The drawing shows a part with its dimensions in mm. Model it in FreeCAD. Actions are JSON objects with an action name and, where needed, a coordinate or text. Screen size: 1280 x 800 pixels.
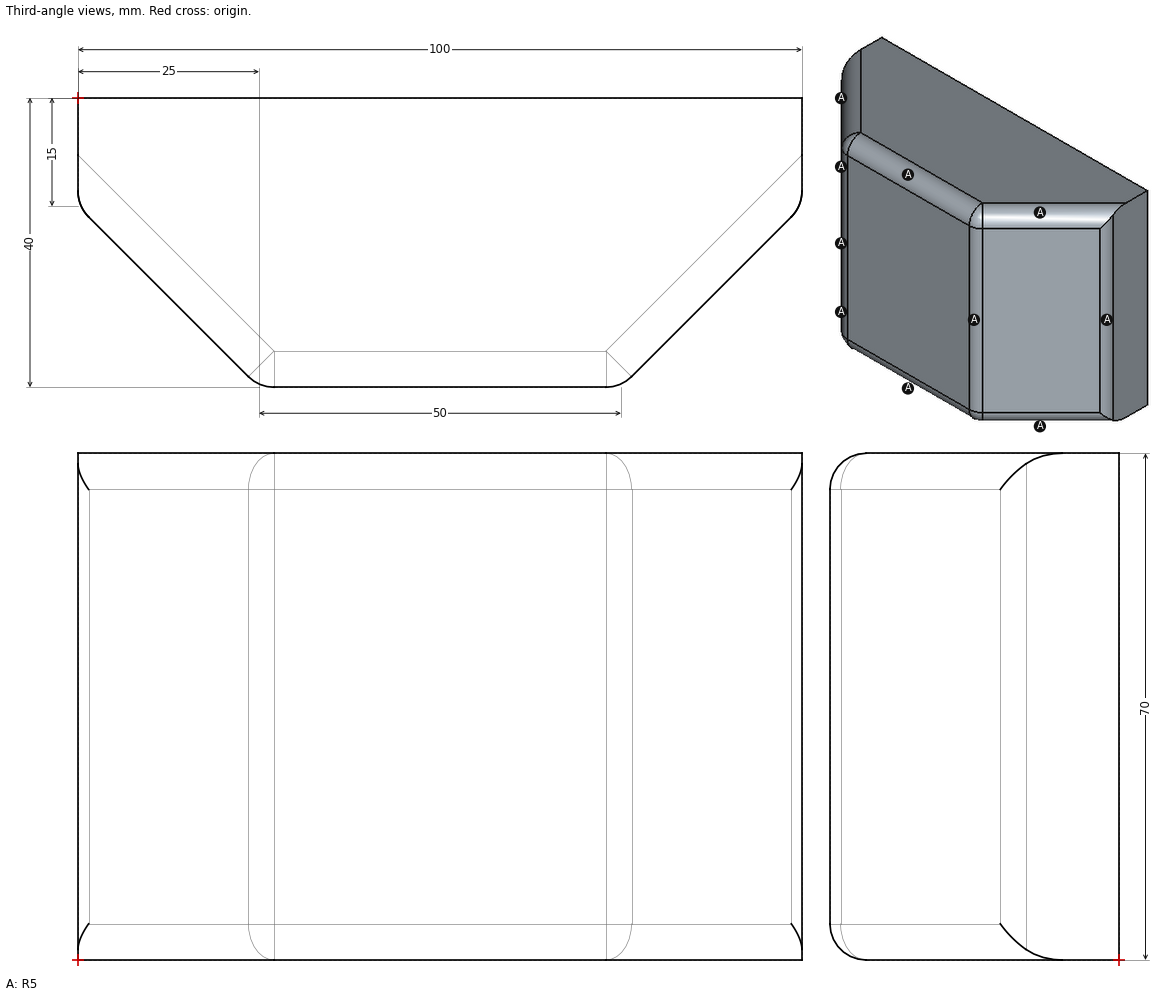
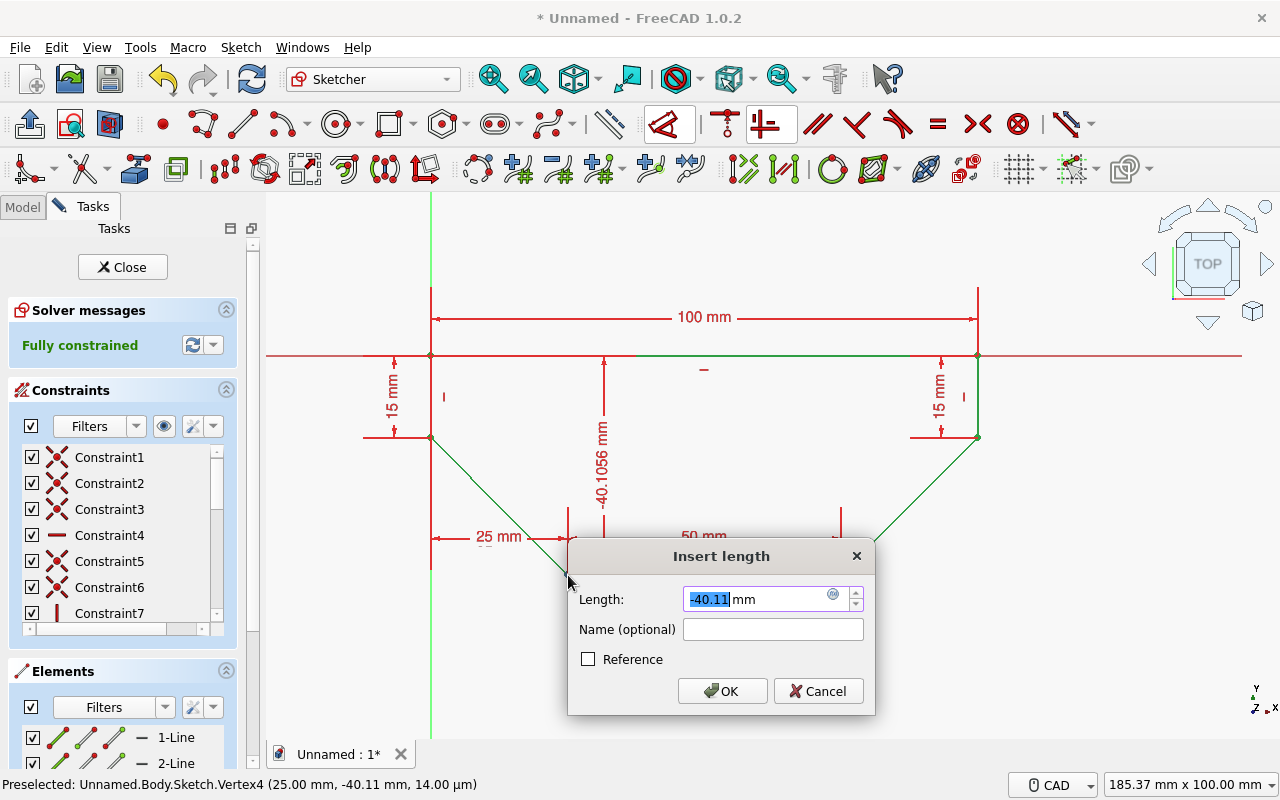
{"action": "type", "text": "-40"}
{"action": "key", "text": "Return"}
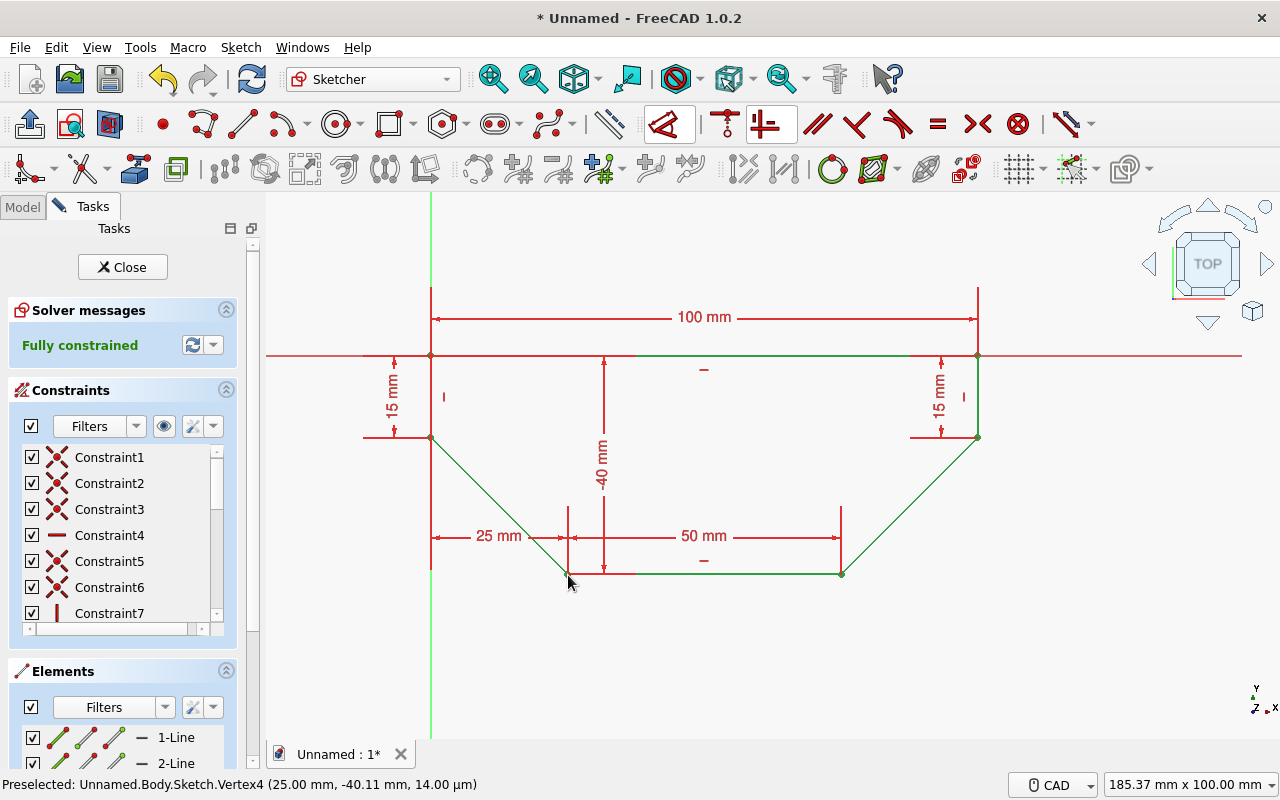
{"action": "left_click", "coordinate": [123, 267]}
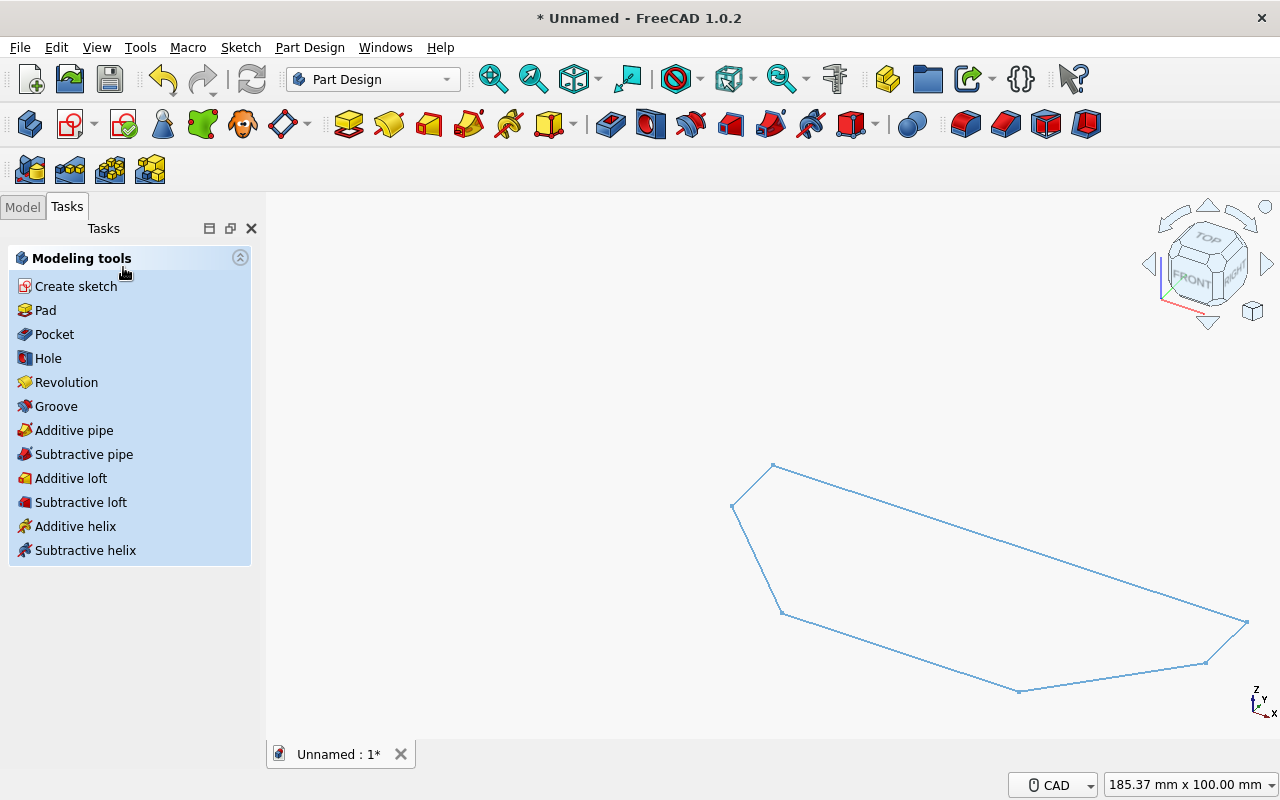
{"action": "left_click", "coordinate": [350, 124]}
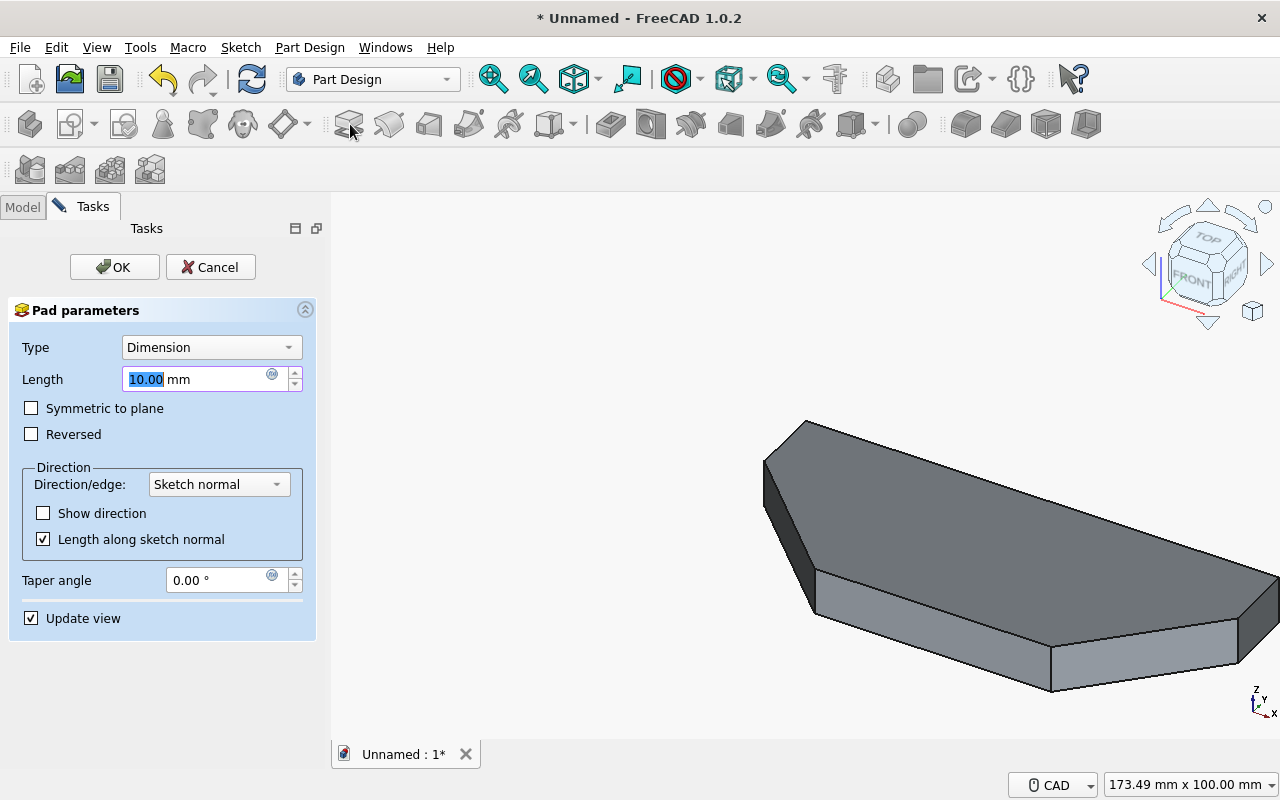
{"action": "type", "text": "70"}
{"action": "key", "text": "Tab"}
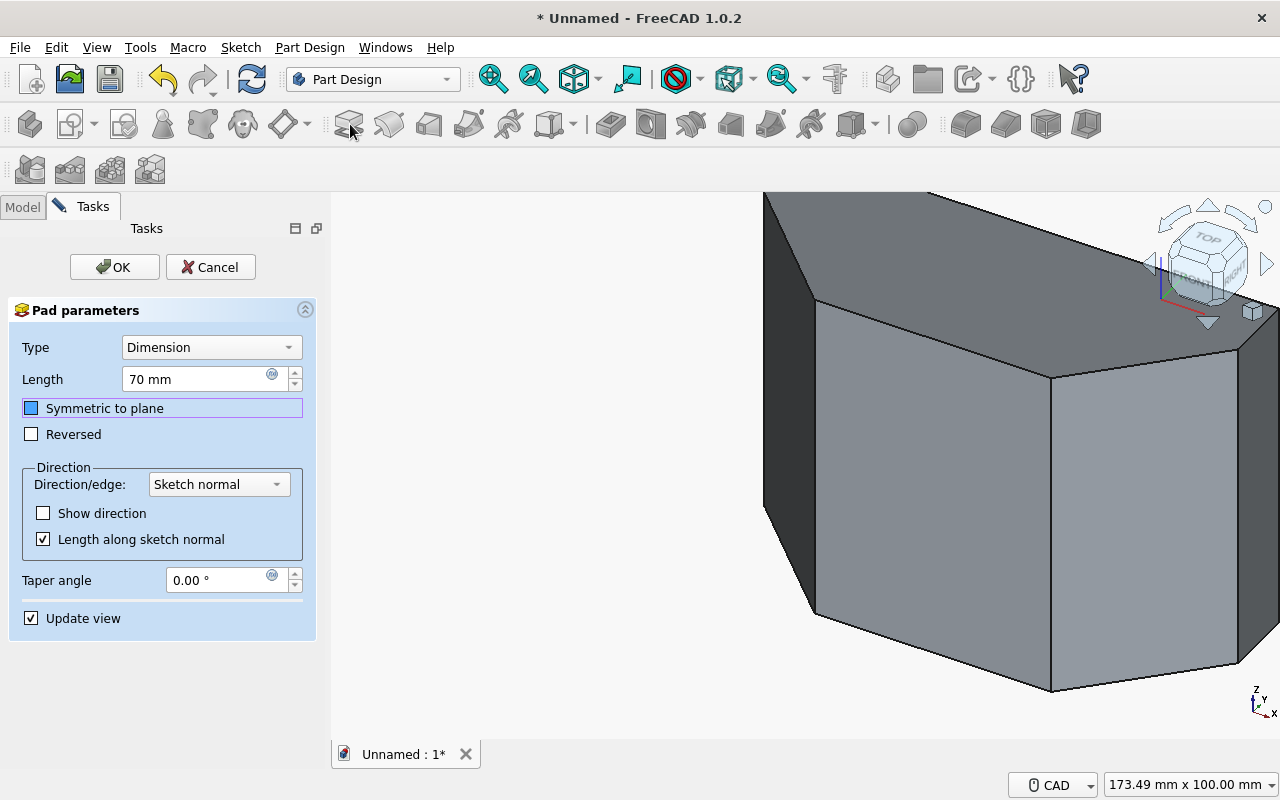
{"action": "left_click", "coordinate": [115, 267]}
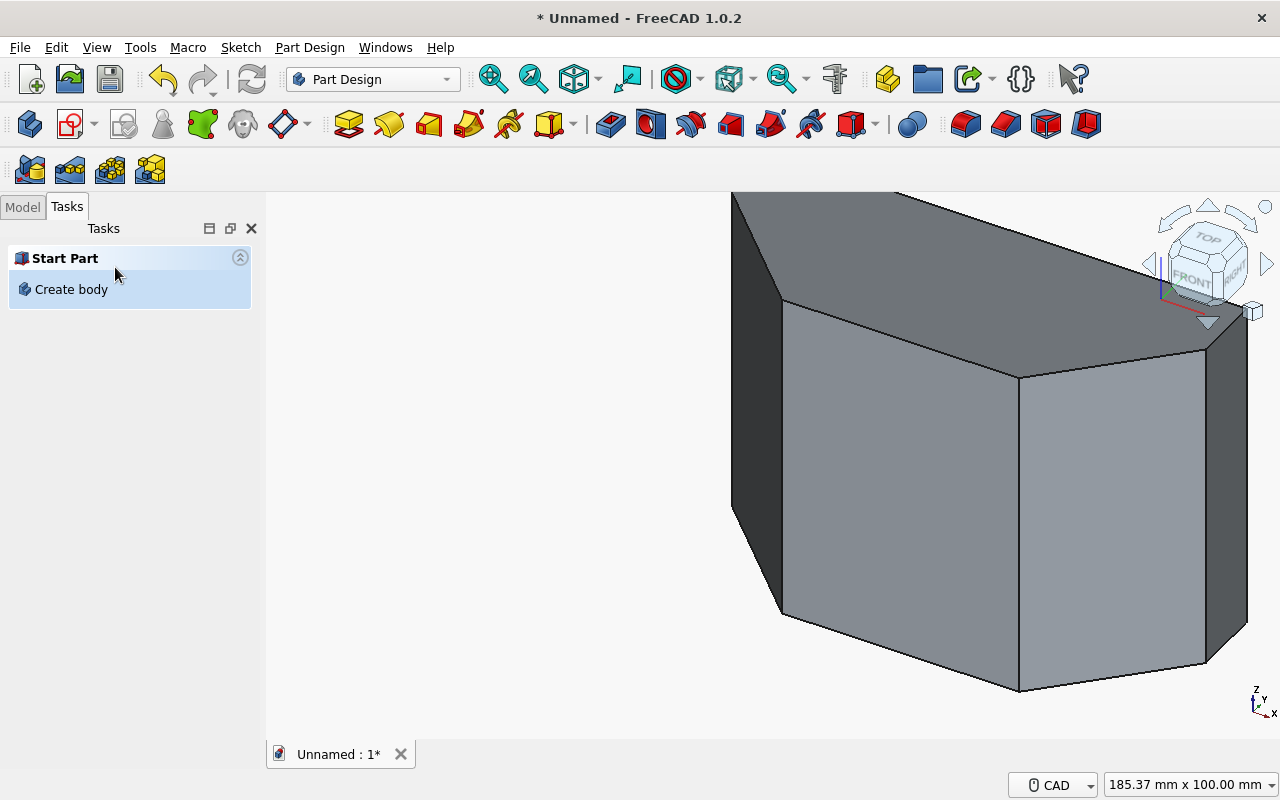
{"action": "left_click", "coordinate": [494, 80]}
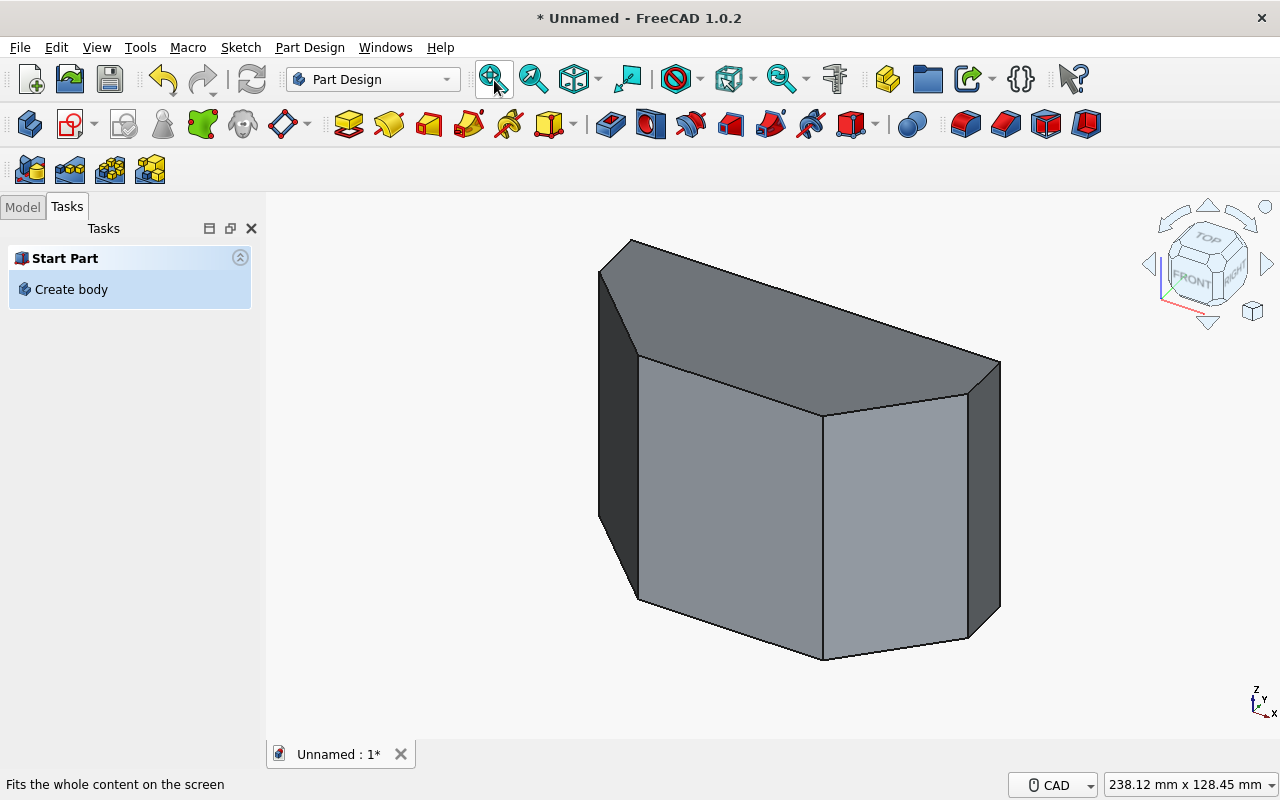
{"action": "left_click", "coordinate": [730, 472]}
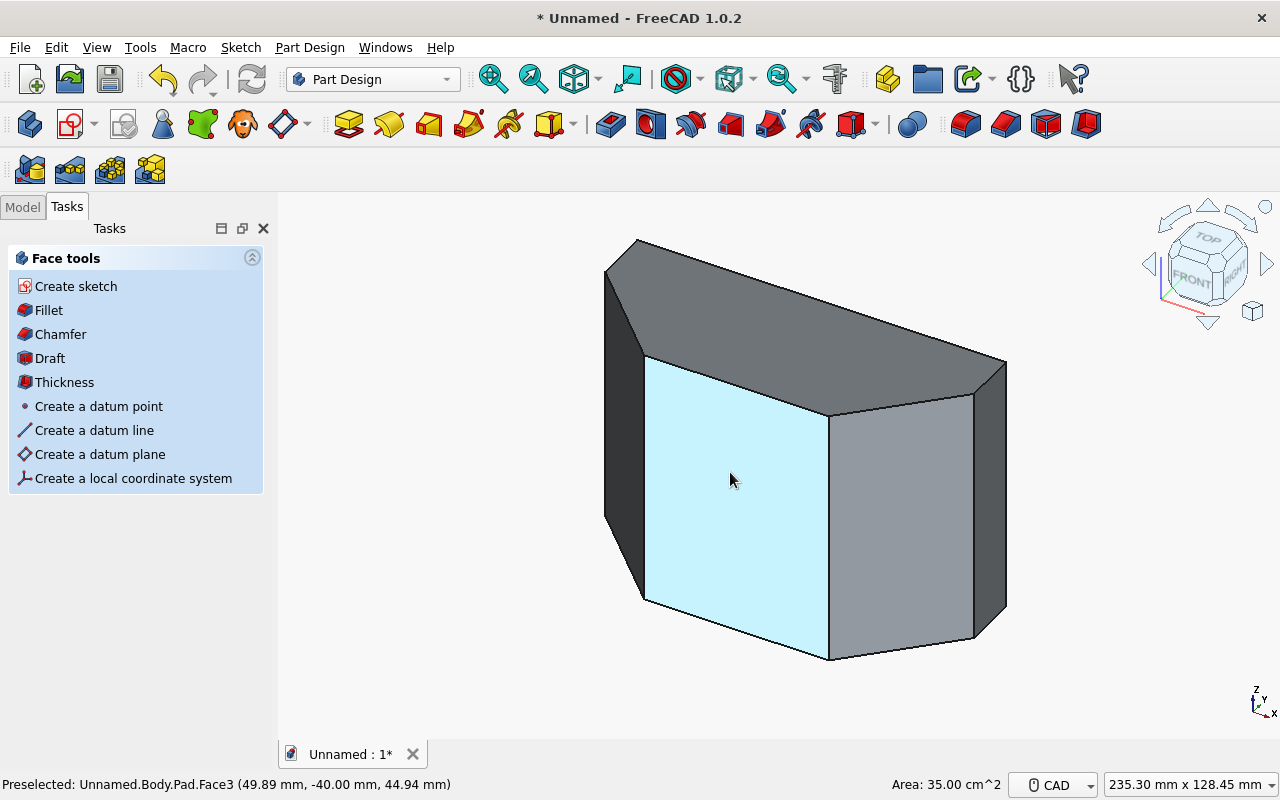
{"action": "left_click", "coordinate": [625, 400], "text": "ctrl"}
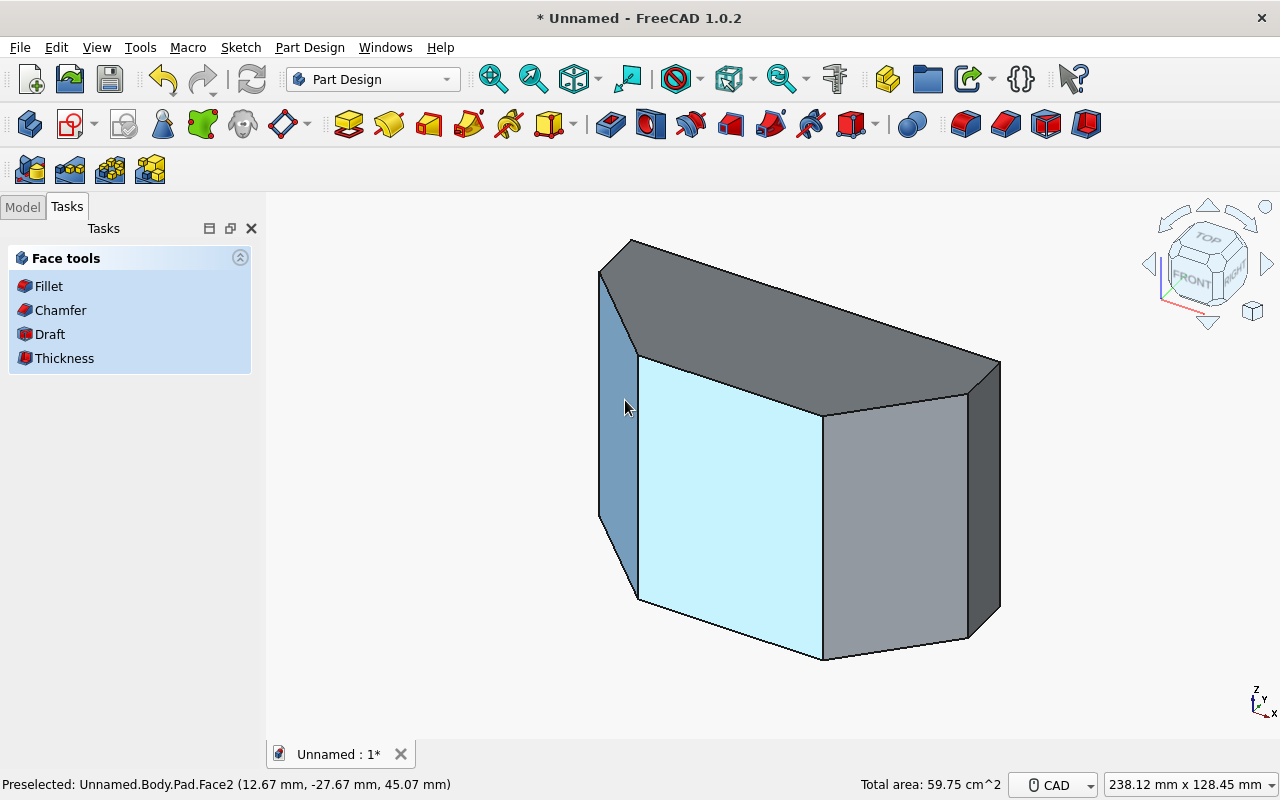
{"action": "left_click", "coordinate": [895, 491], "text": "ctrl"}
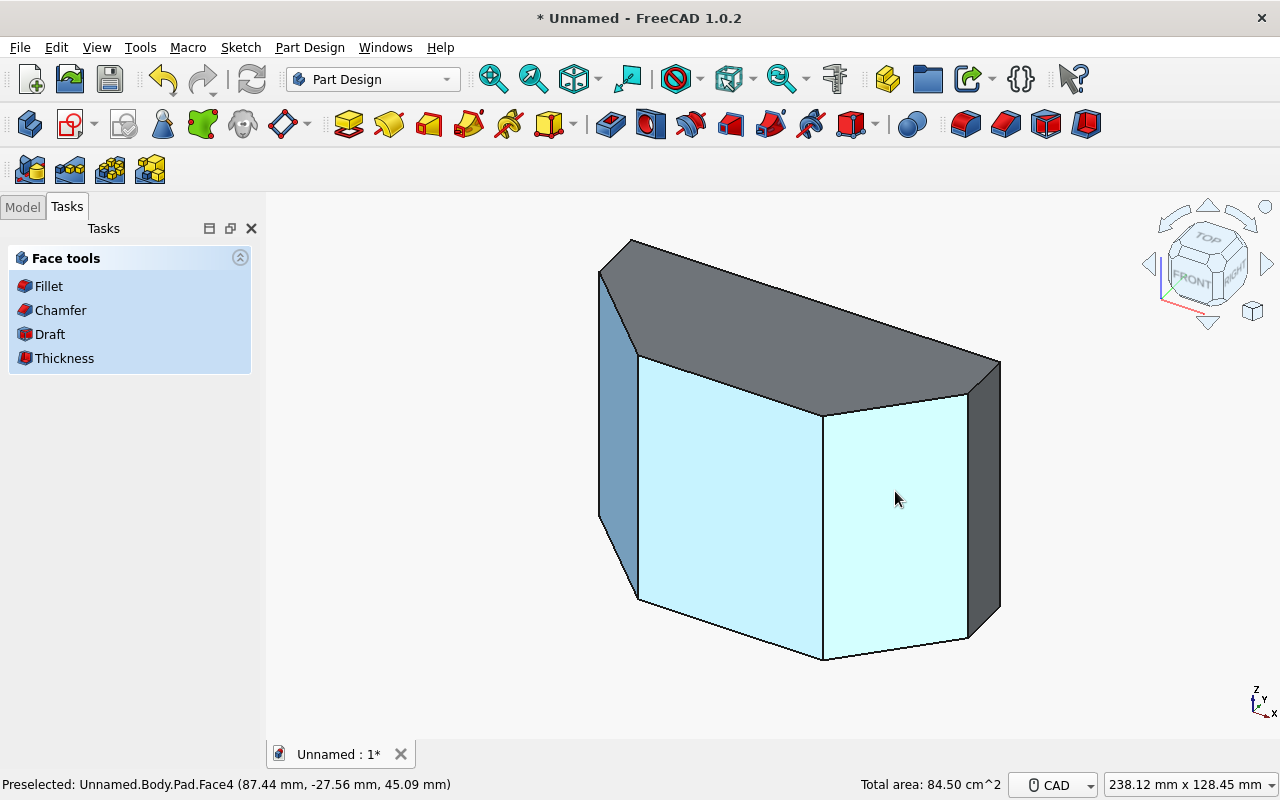
{"action": "left_click", "coordinate": [966, 124]}